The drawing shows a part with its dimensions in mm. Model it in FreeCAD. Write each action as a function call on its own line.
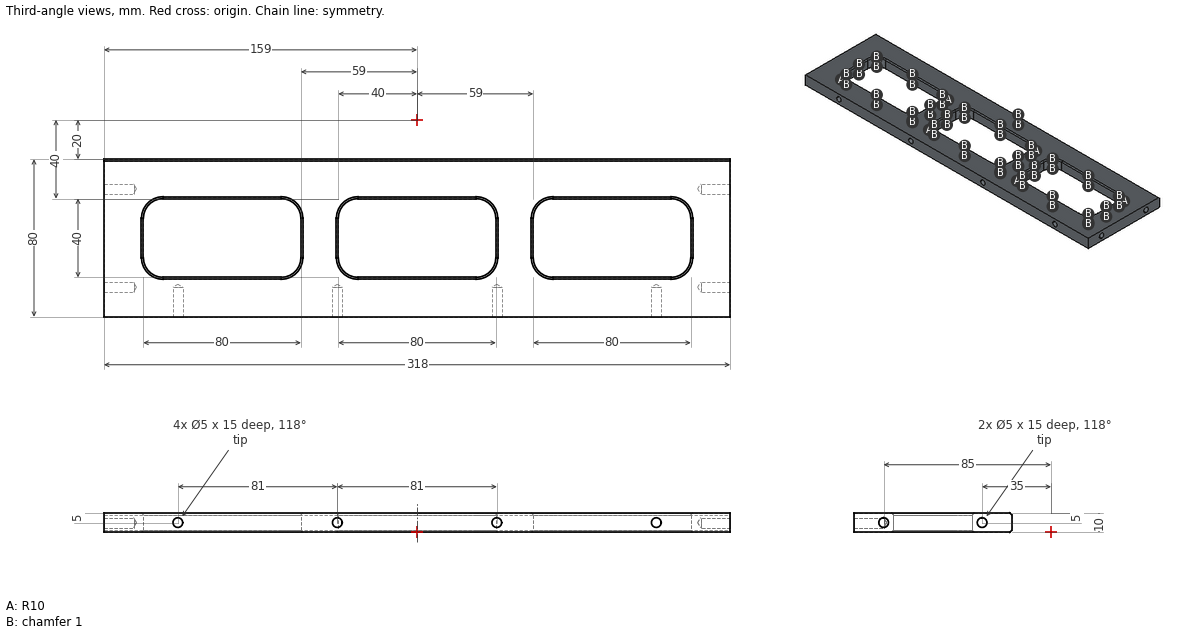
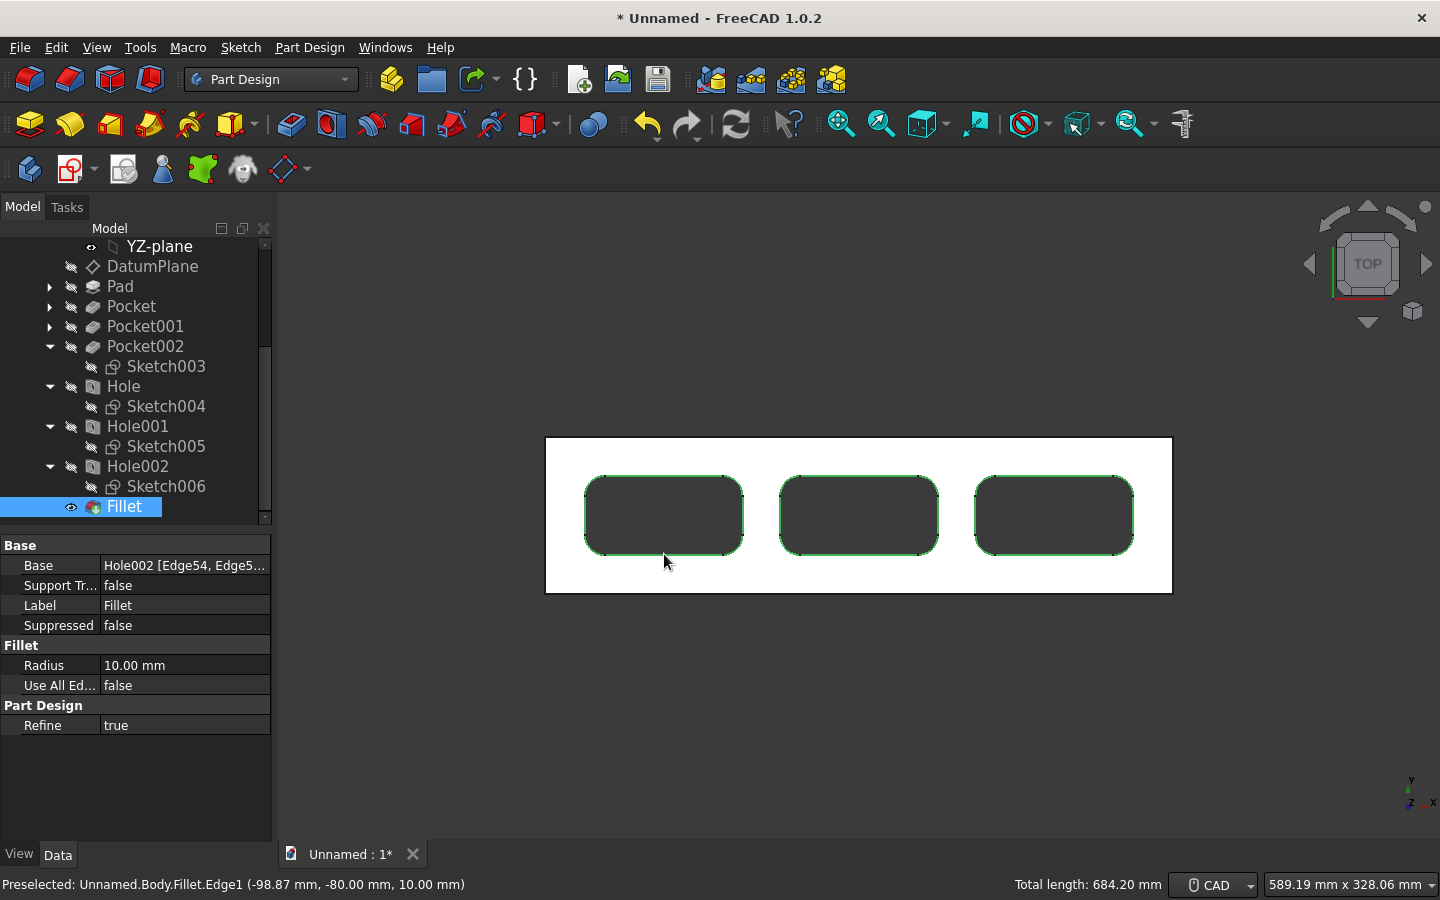
click(859, 436, ctrl)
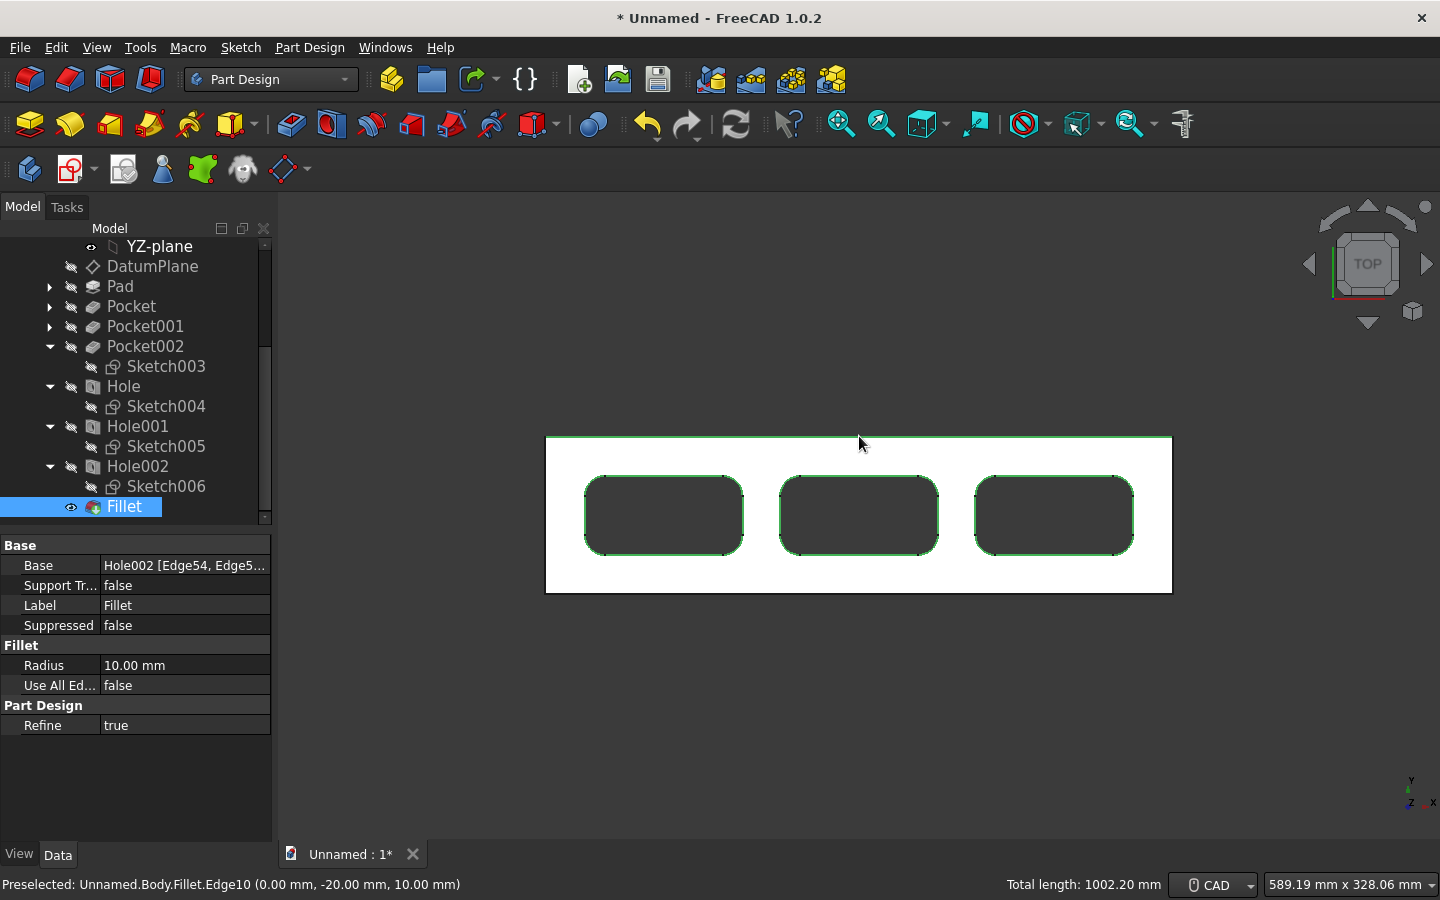
key(0)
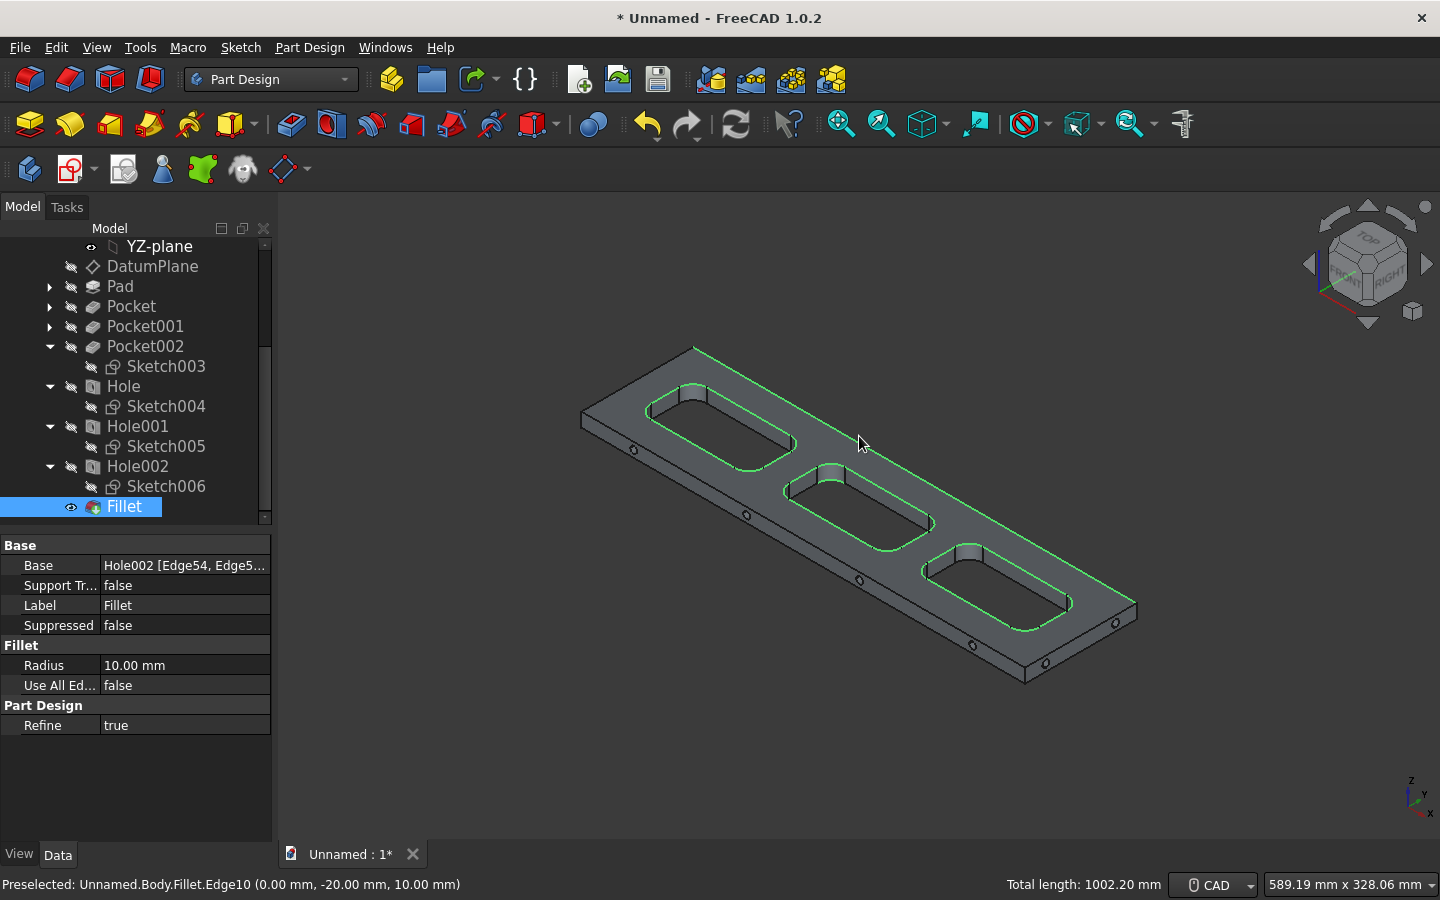
key(1)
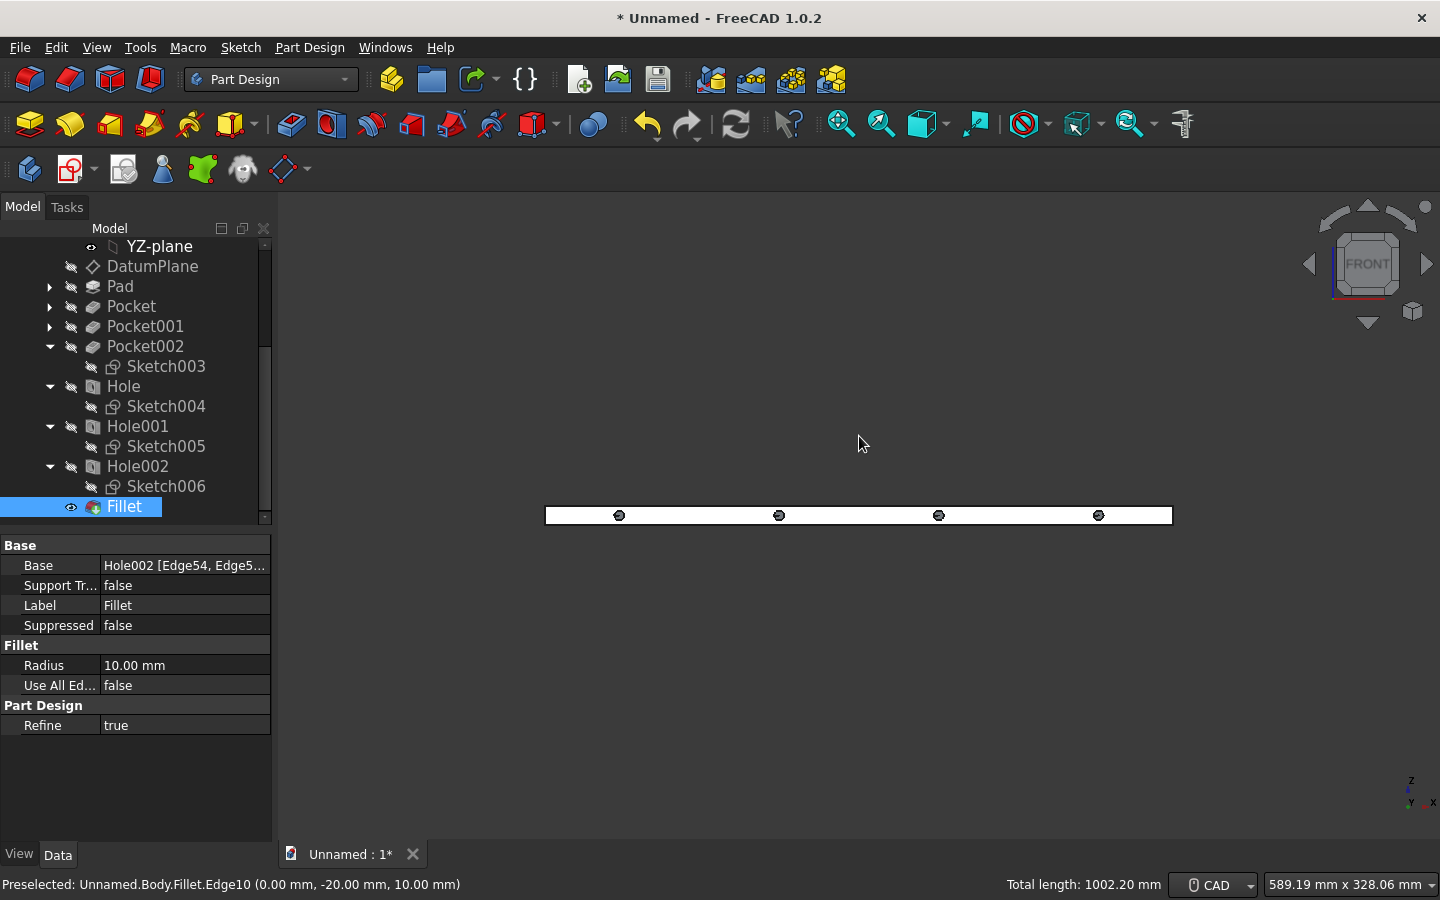
key(3)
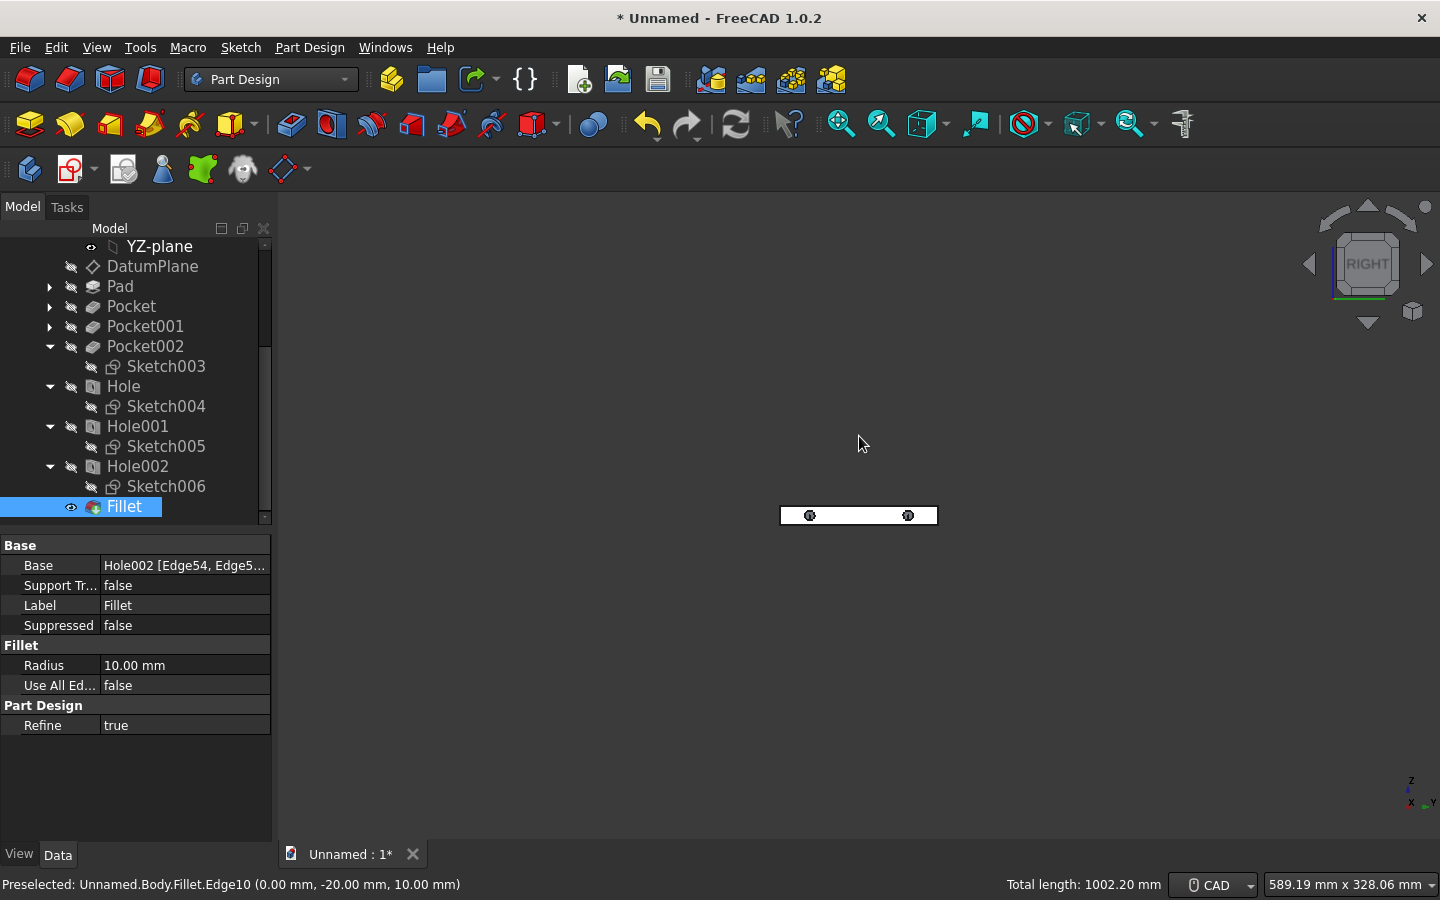
click(842, 124)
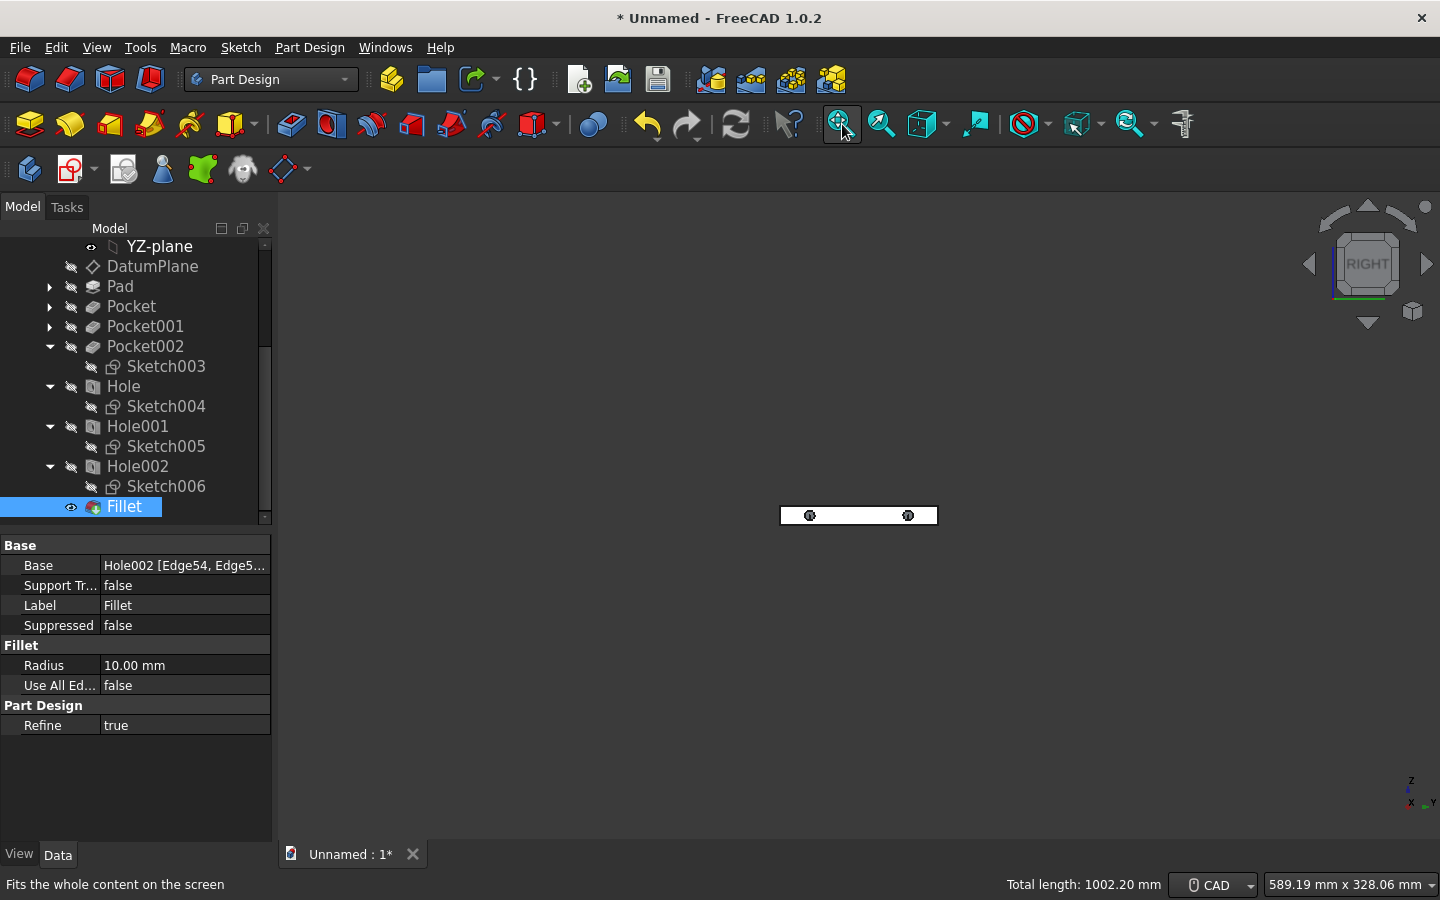
key(5)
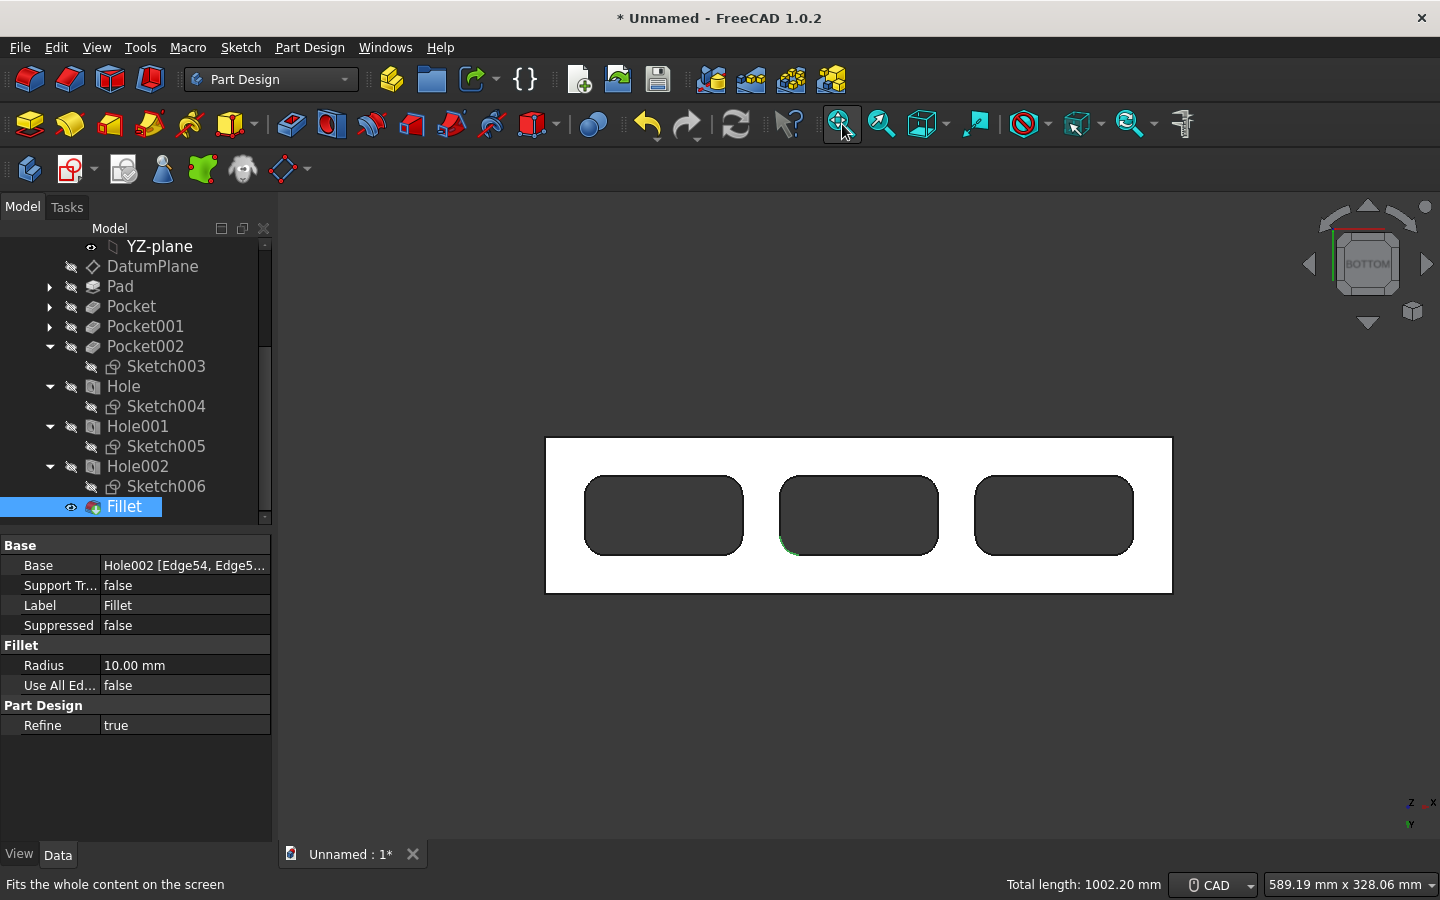
click(859, 554, ctrl)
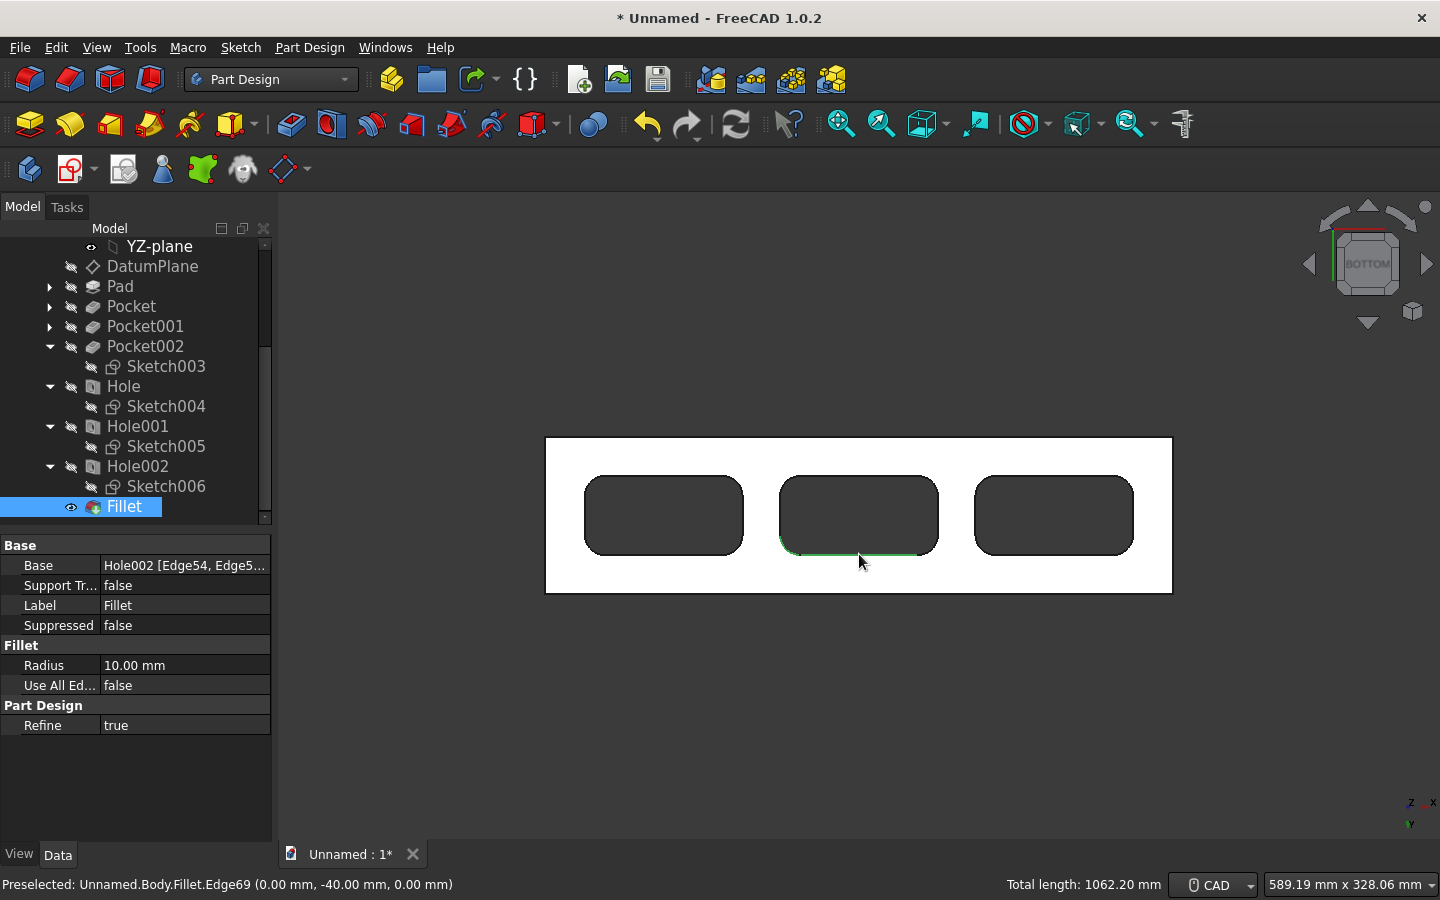
click(938, 514, ctrl)